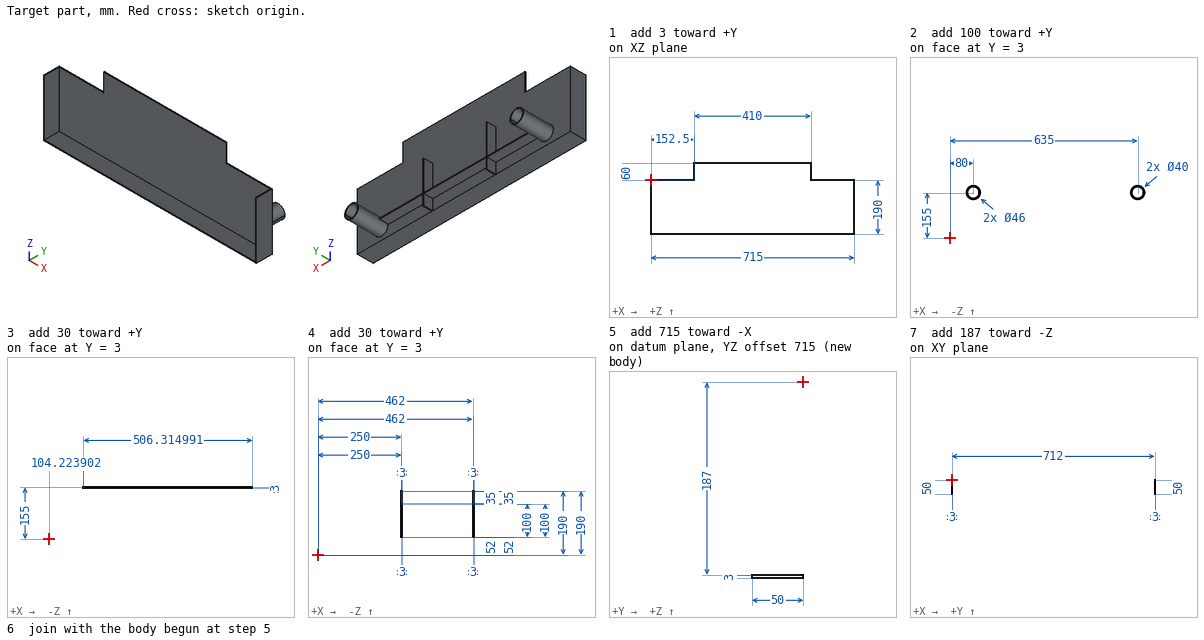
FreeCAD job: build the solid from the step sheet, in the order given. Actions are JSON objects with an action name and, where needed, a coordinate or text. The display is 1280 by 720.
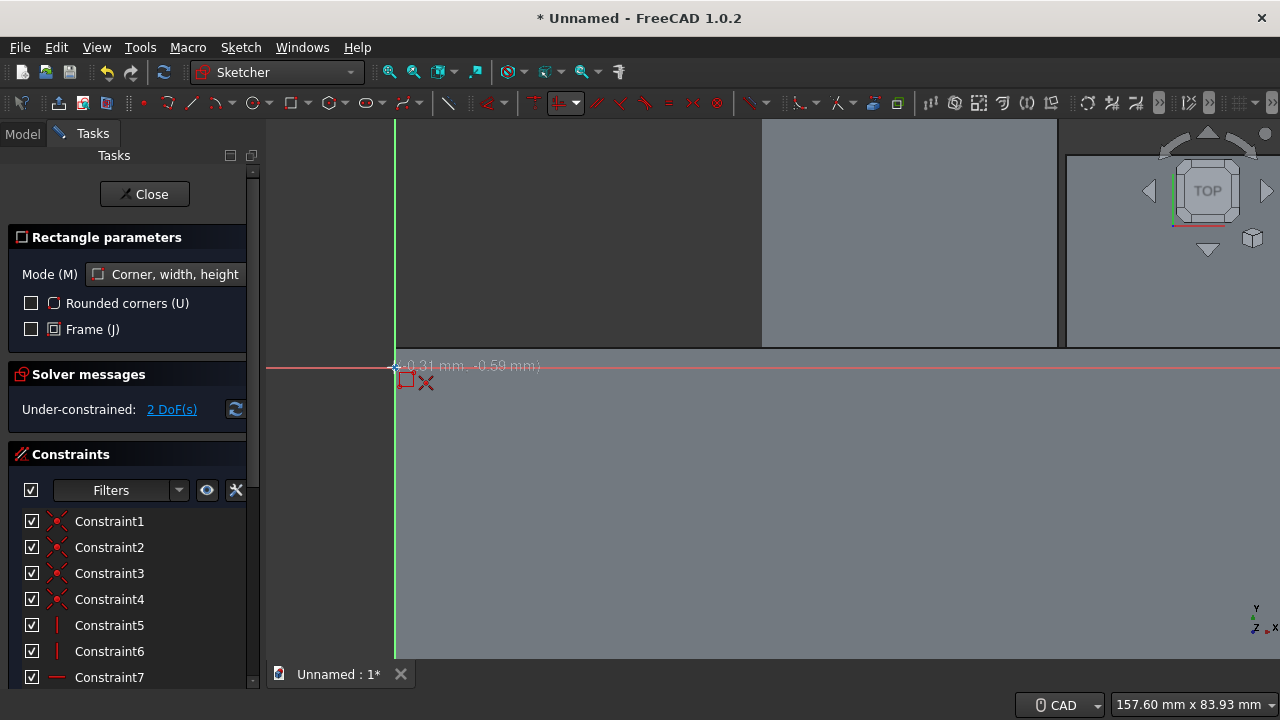
{"action": "scroll", "coordinate": [393, 367], "scroll_direction": "down", "scroll_amount": 10}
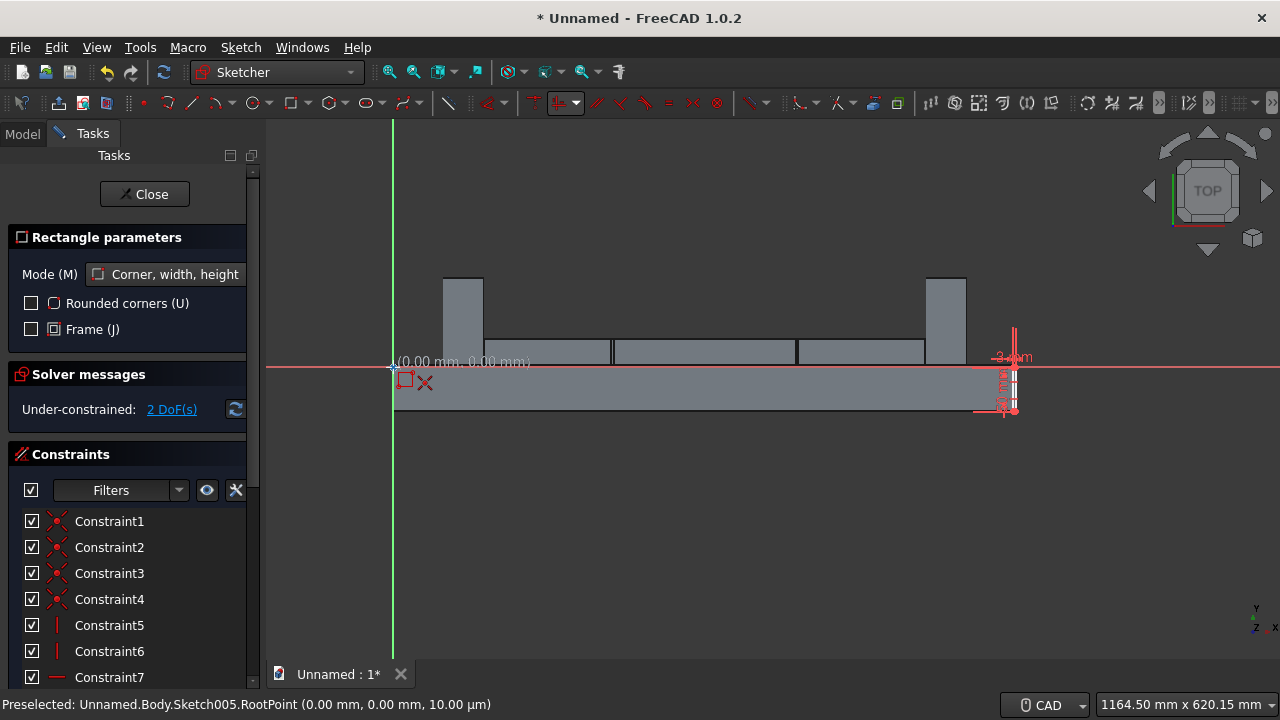
{"action": "left_click", "coordinate": [393, 367]}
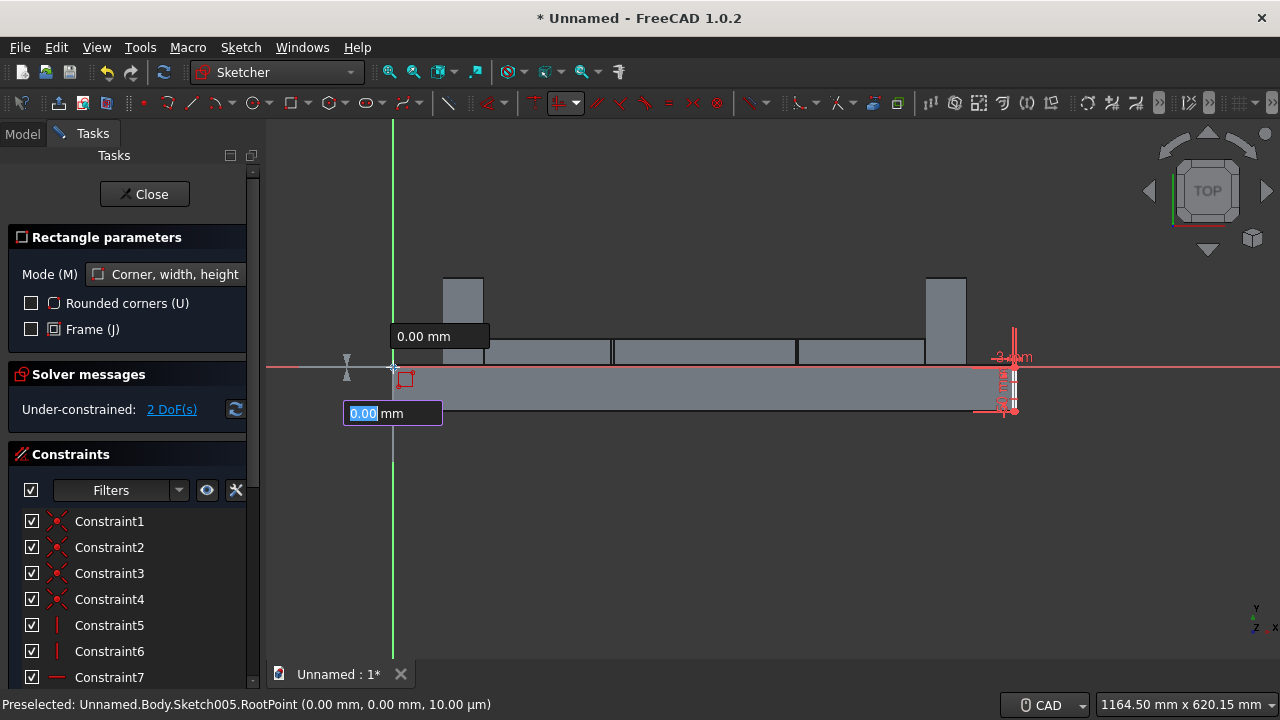
{"action": "scroll", "coordinate": [396, 411], "scroll_direction": "up", "scroll_amount": 10}
{"action": "mouse_move", "coordinate": [395, 408]}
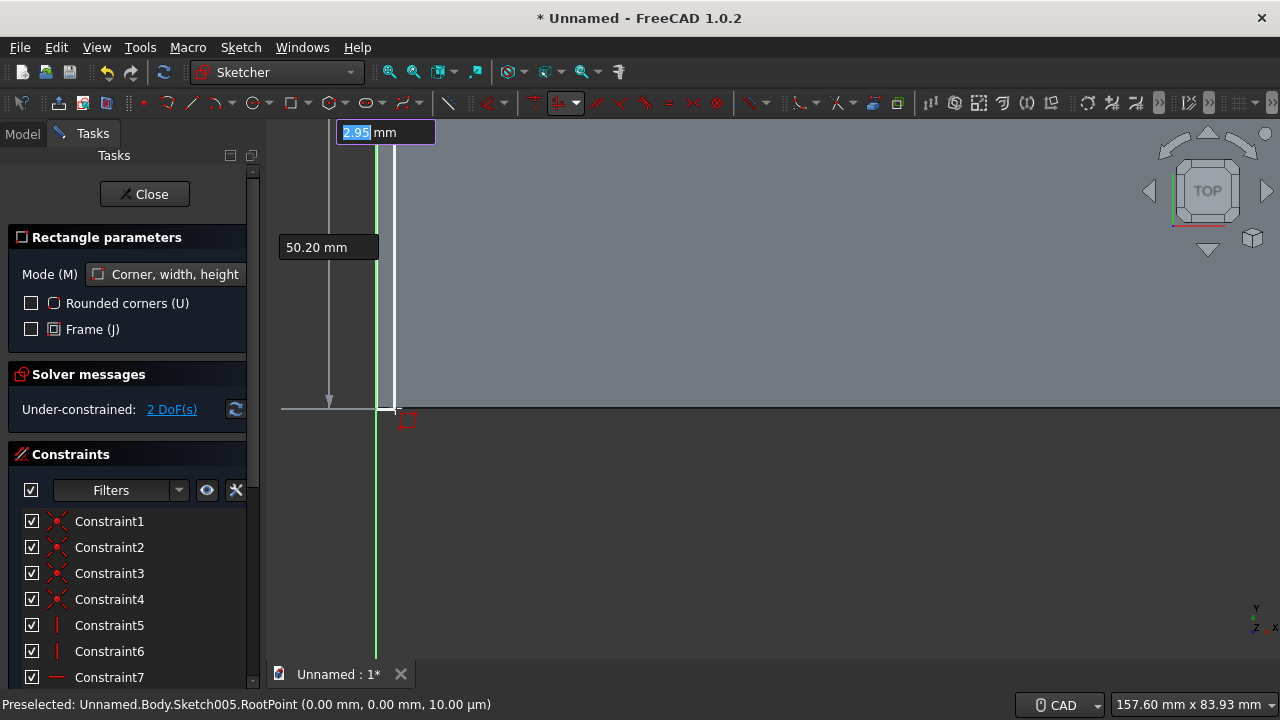
{"action": "type", "text": "3"}
{"action": "key", "text": "Tab"}
{"action": "type", "text": "50"}
{"action": "key", "text": "Return"}
{"action": "key", "text": "Escape"}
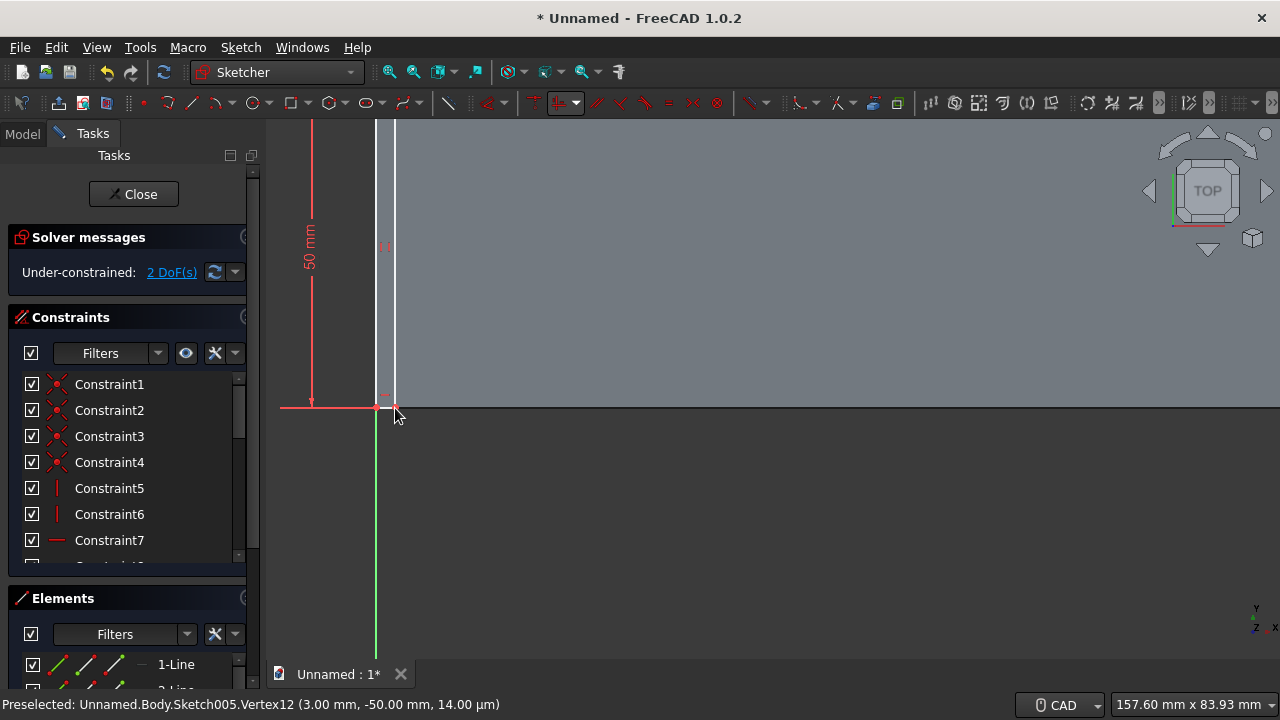
{"action": "scroll", "coordinate": [396, 411], "scroll_direction": "down", "scroll_amount": 10}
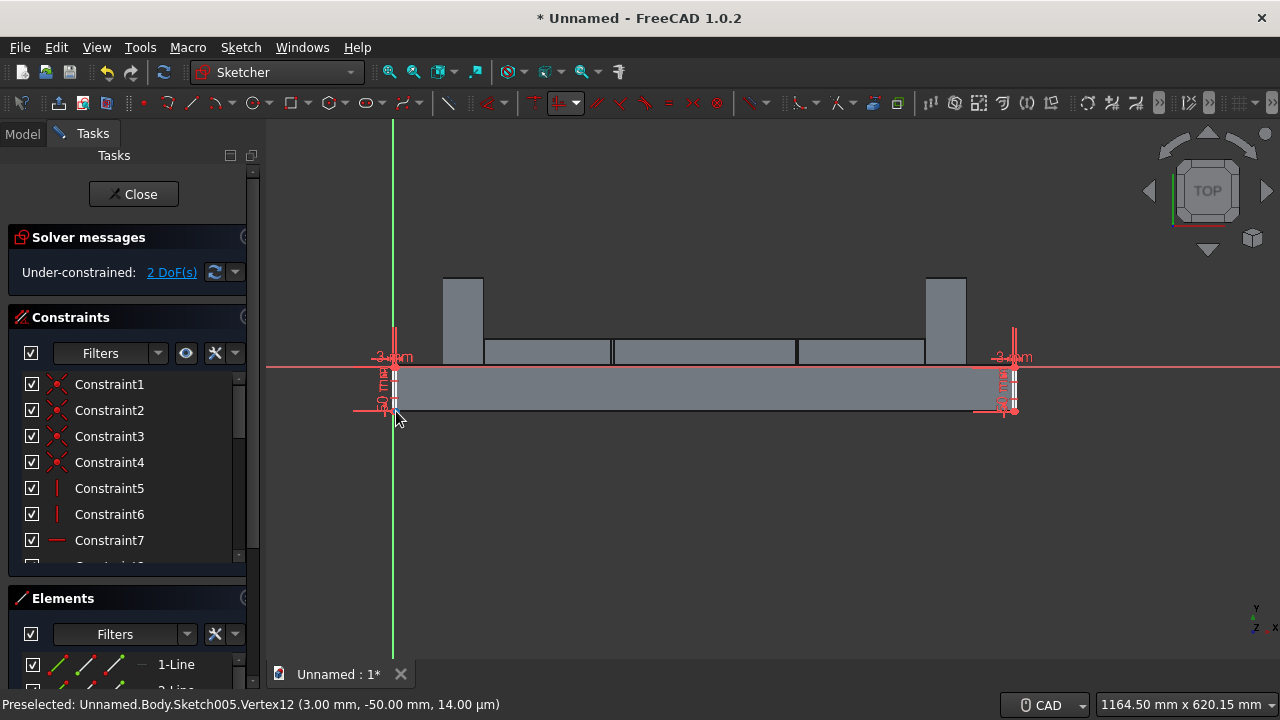
{"action": "scroll", "coordinate": [1013, 368], "scroll_direction": "up", "scroll_amount": 8}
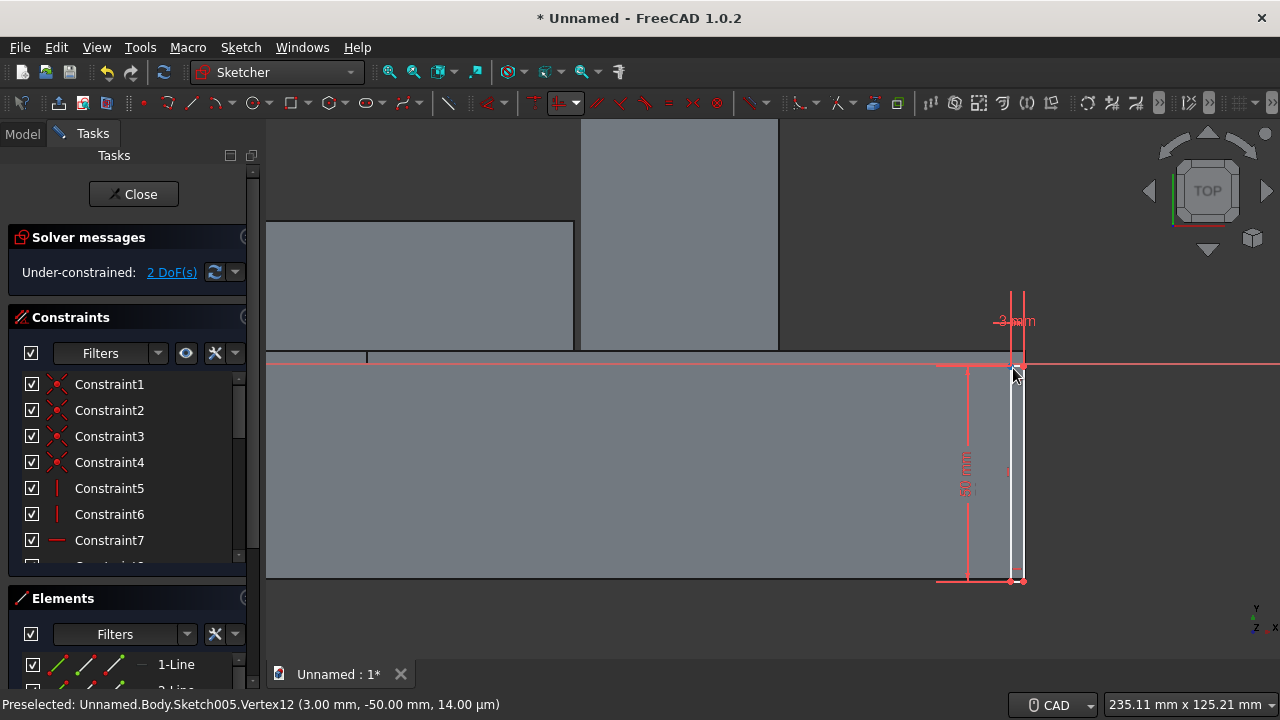
{"action": "left_click", "coordinate": [1011, 366]}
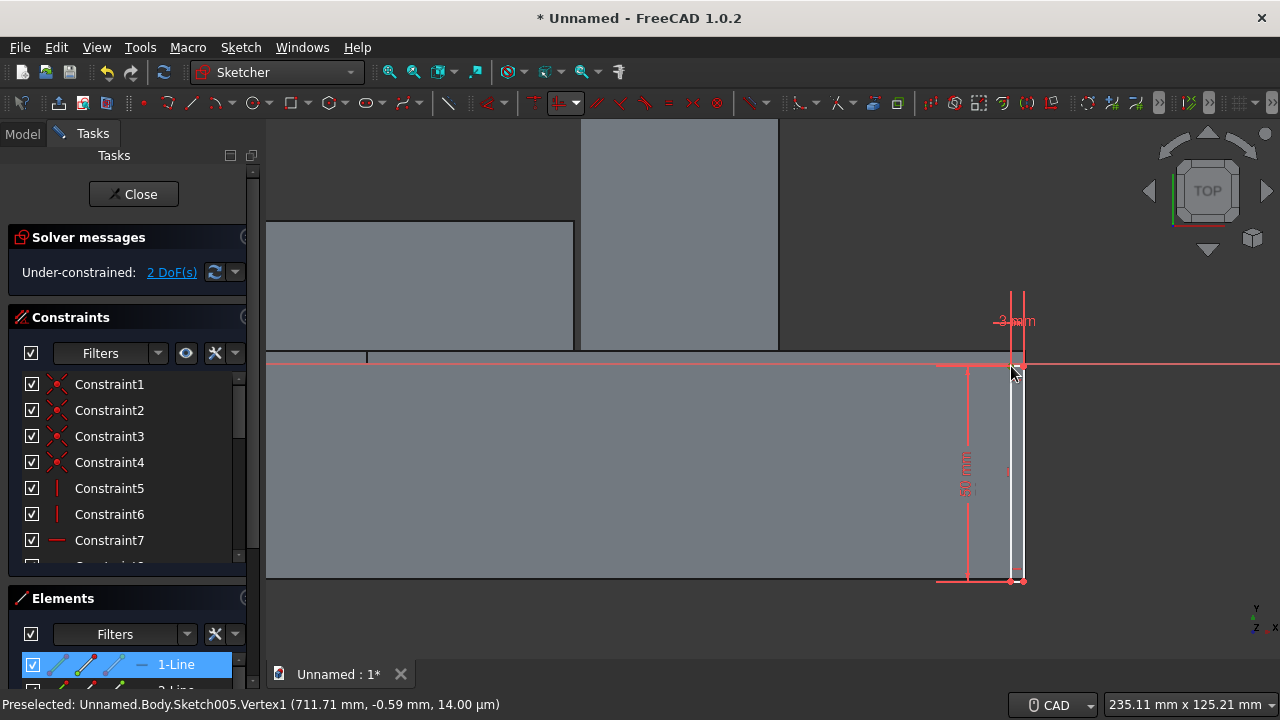
{"action": "left_click", "coordinate": [353, 364]}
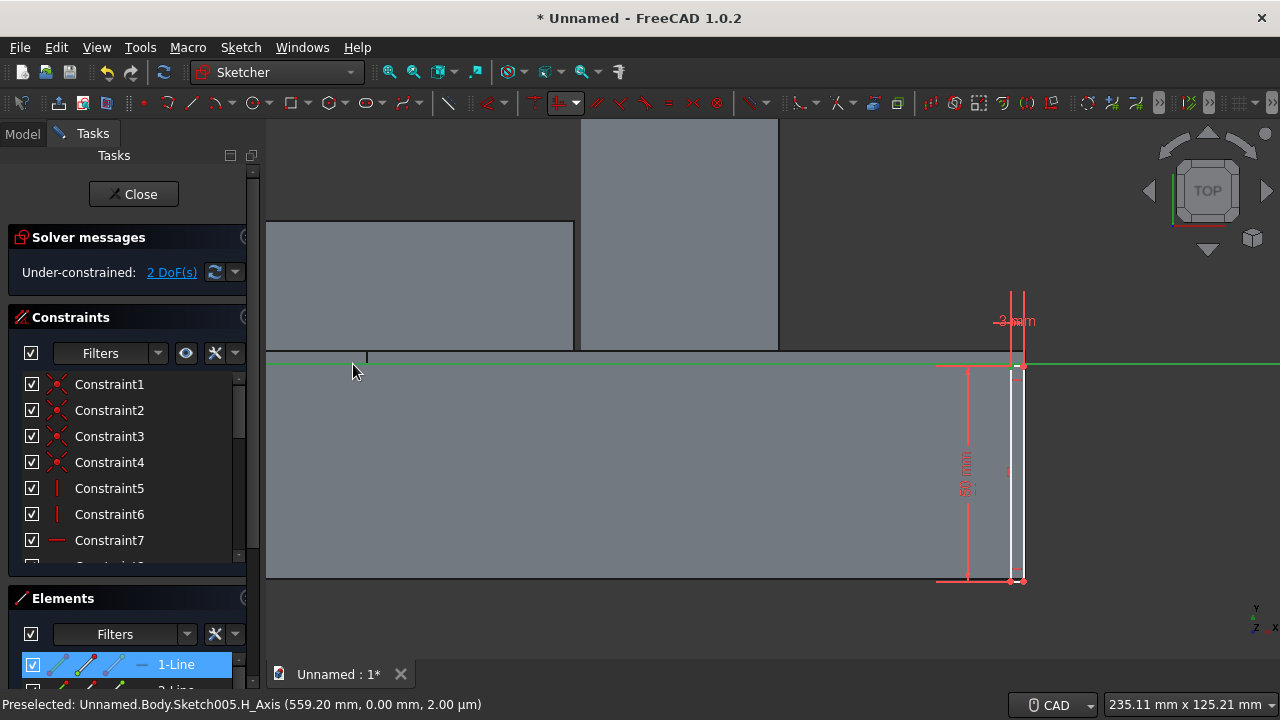
{"action": "left_click", "coordinate": [534, 104]}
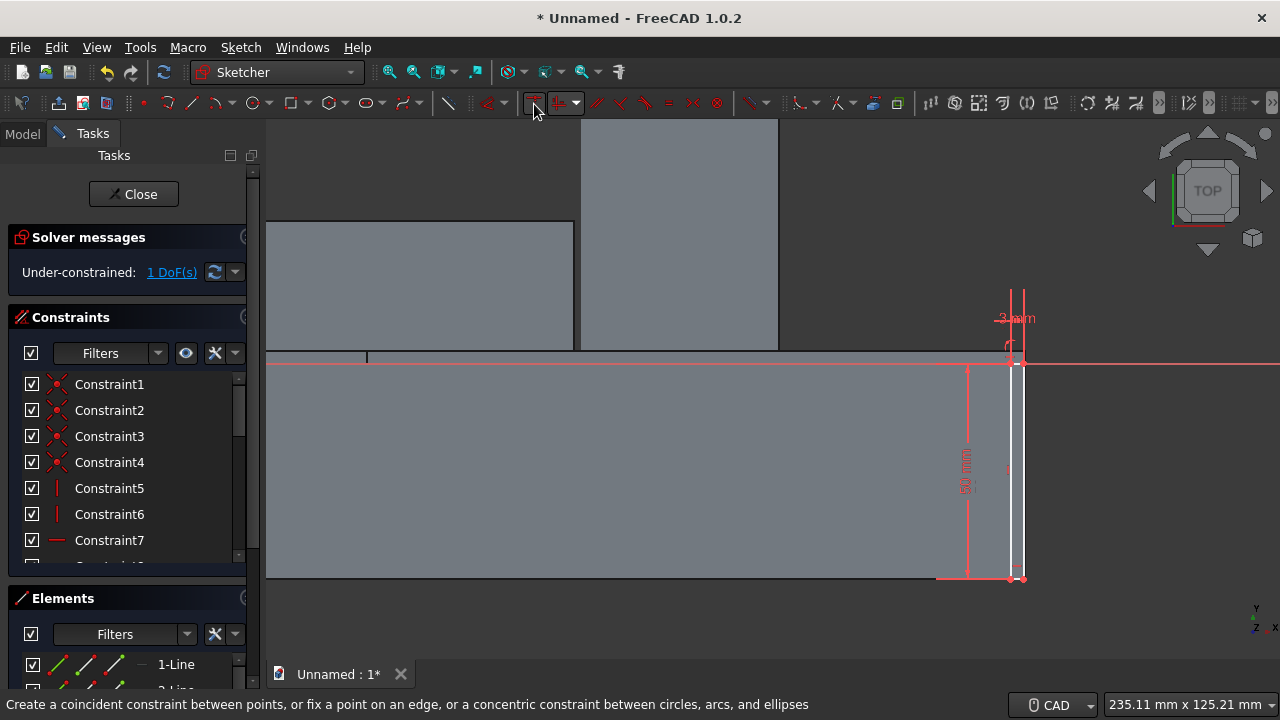
{"action": "left_click", "coordinate": [488, 104]}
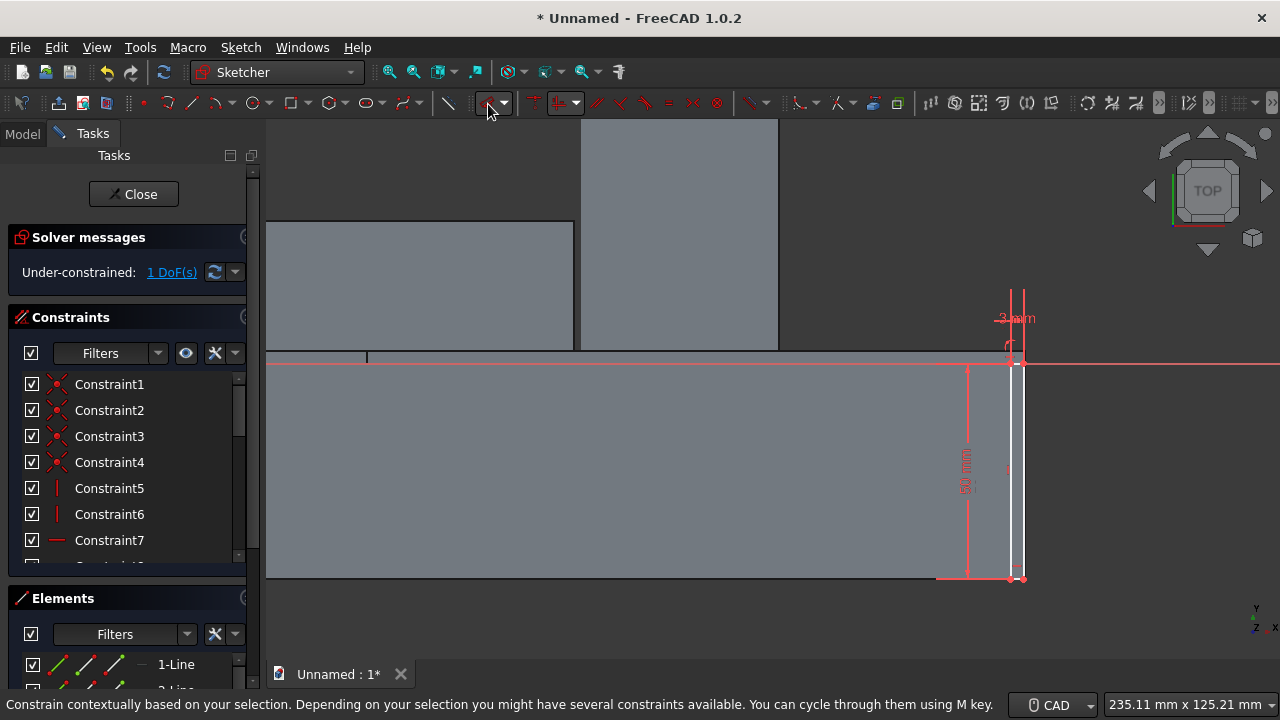
{"action": "left_click", "coordinate": [1011, 364]}
{"action": "left_click", "coordinate": [652, 330]}